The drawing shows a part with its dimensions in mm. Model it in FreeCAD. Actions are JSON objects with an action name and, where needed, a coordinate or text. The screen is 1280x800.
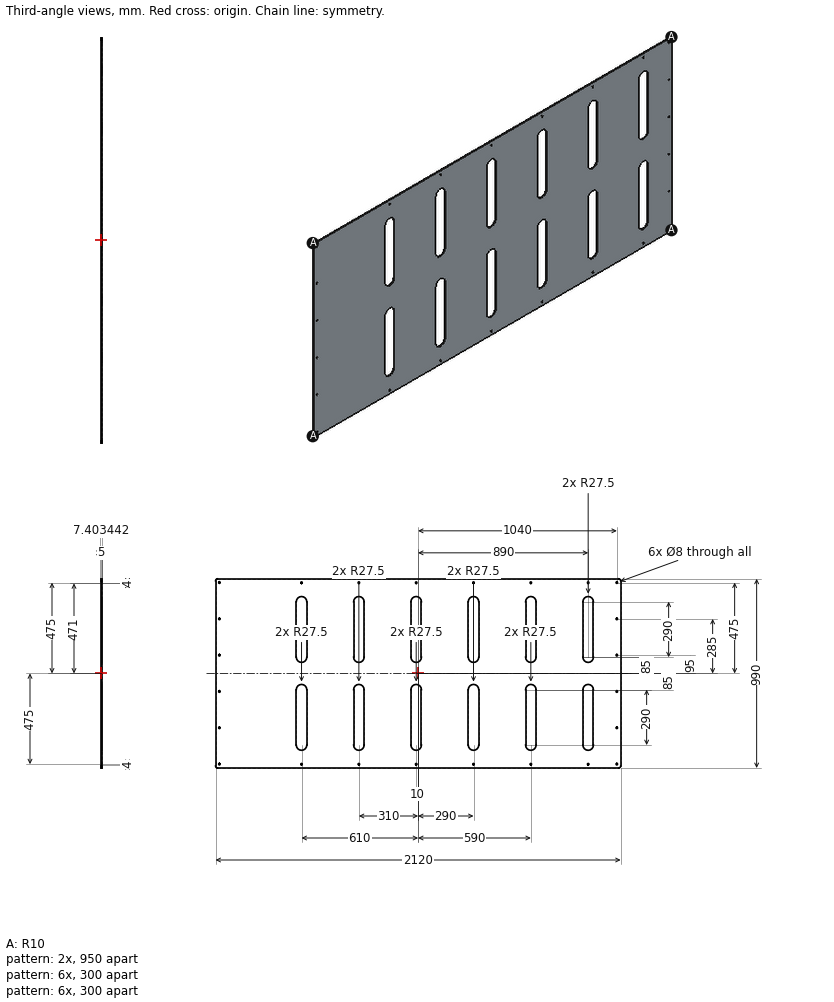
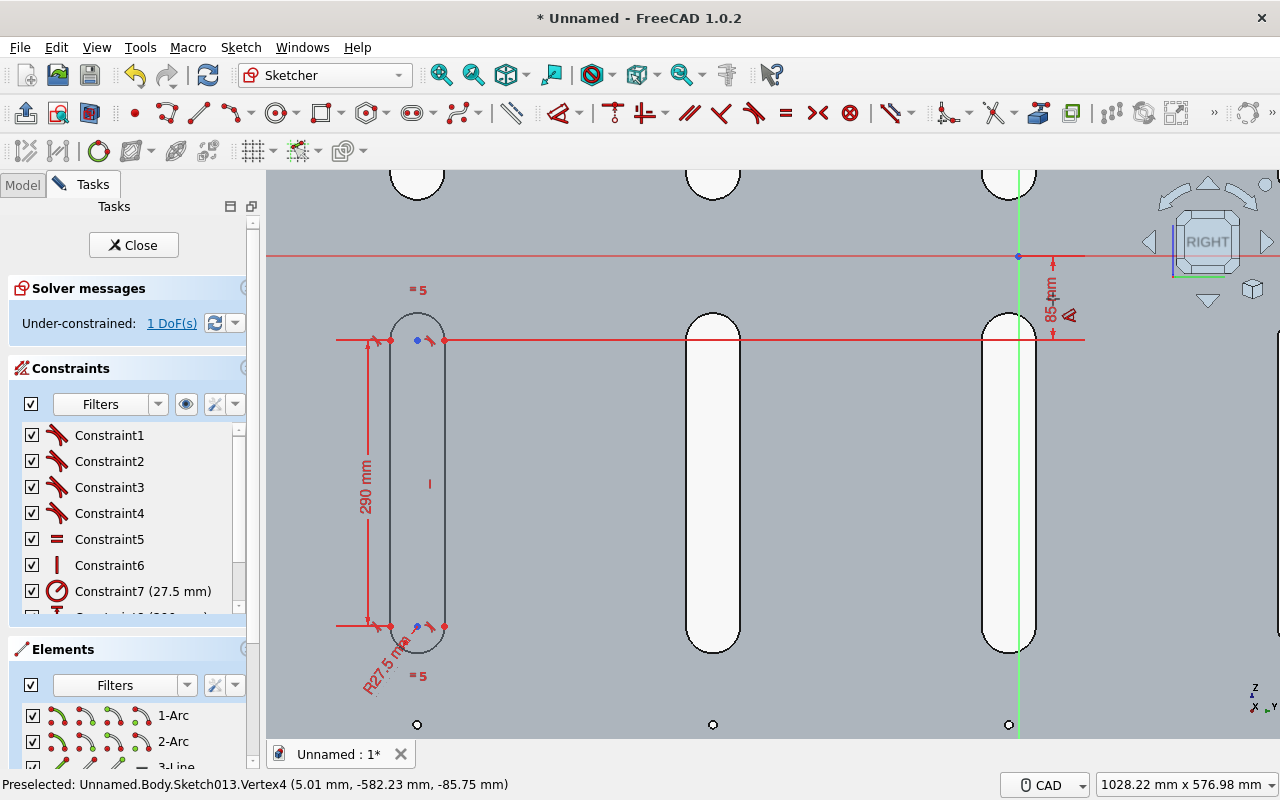
{"action": "left_click", "coordinate": [417, 626]}
{"action": "left_click", "coordinate": [718, 222]}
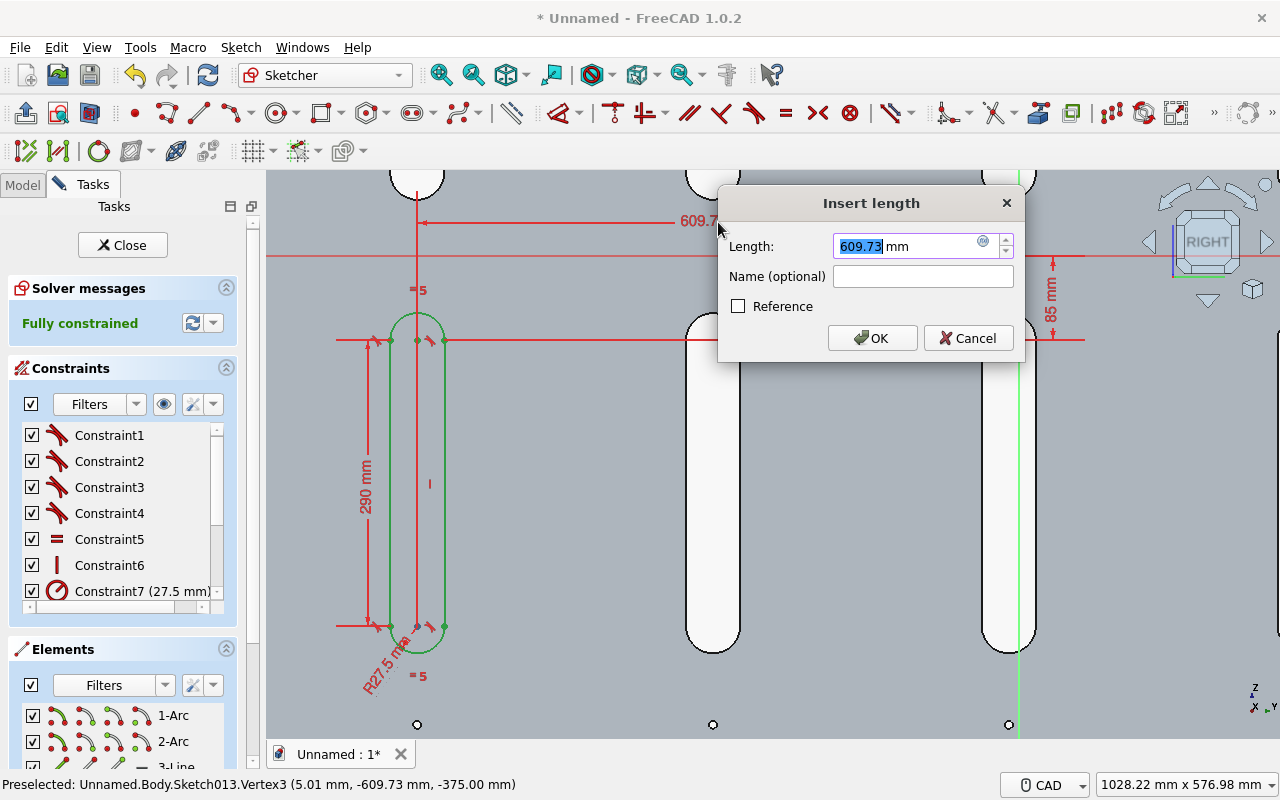
{"action": "type", "text": "610"}
{"action": "key", "text": "Return"}
{"action": "key", "text": "Escape"}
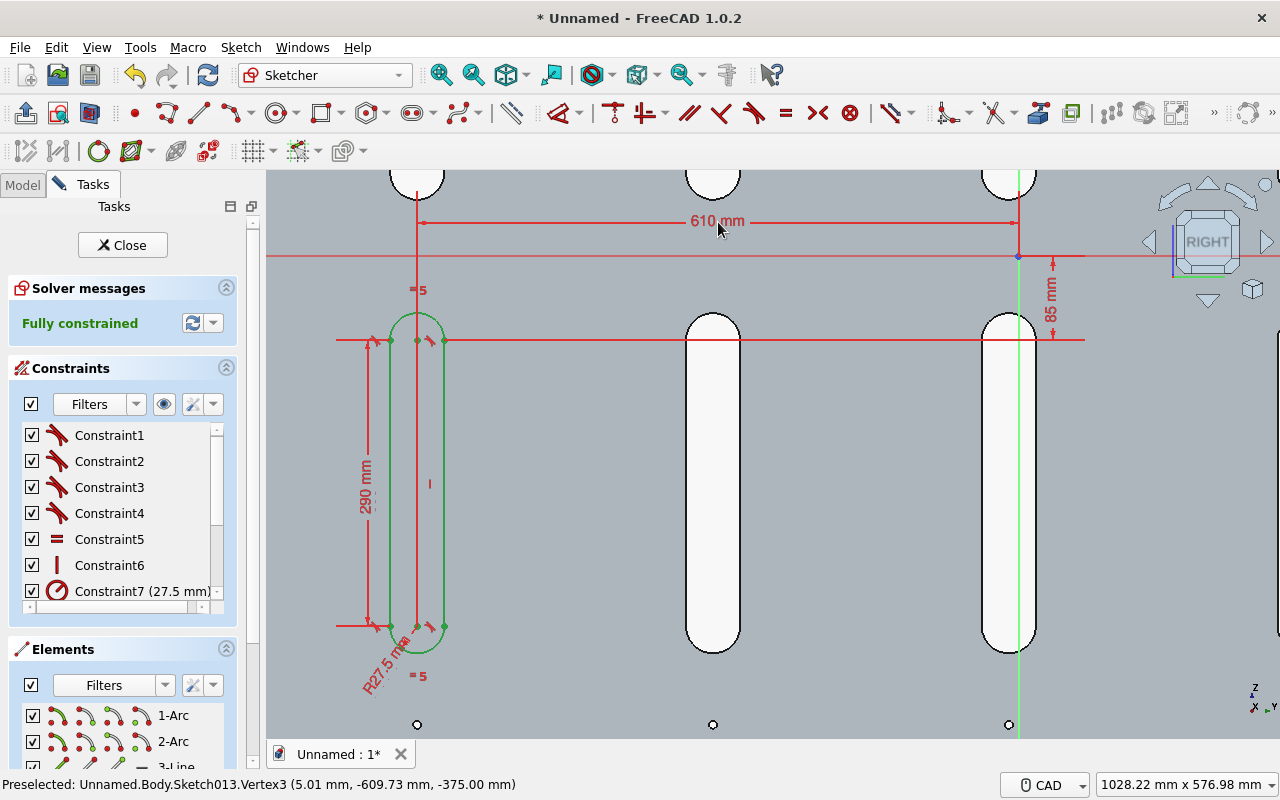
{"action": "left_click", "coordinate": [123, 245]}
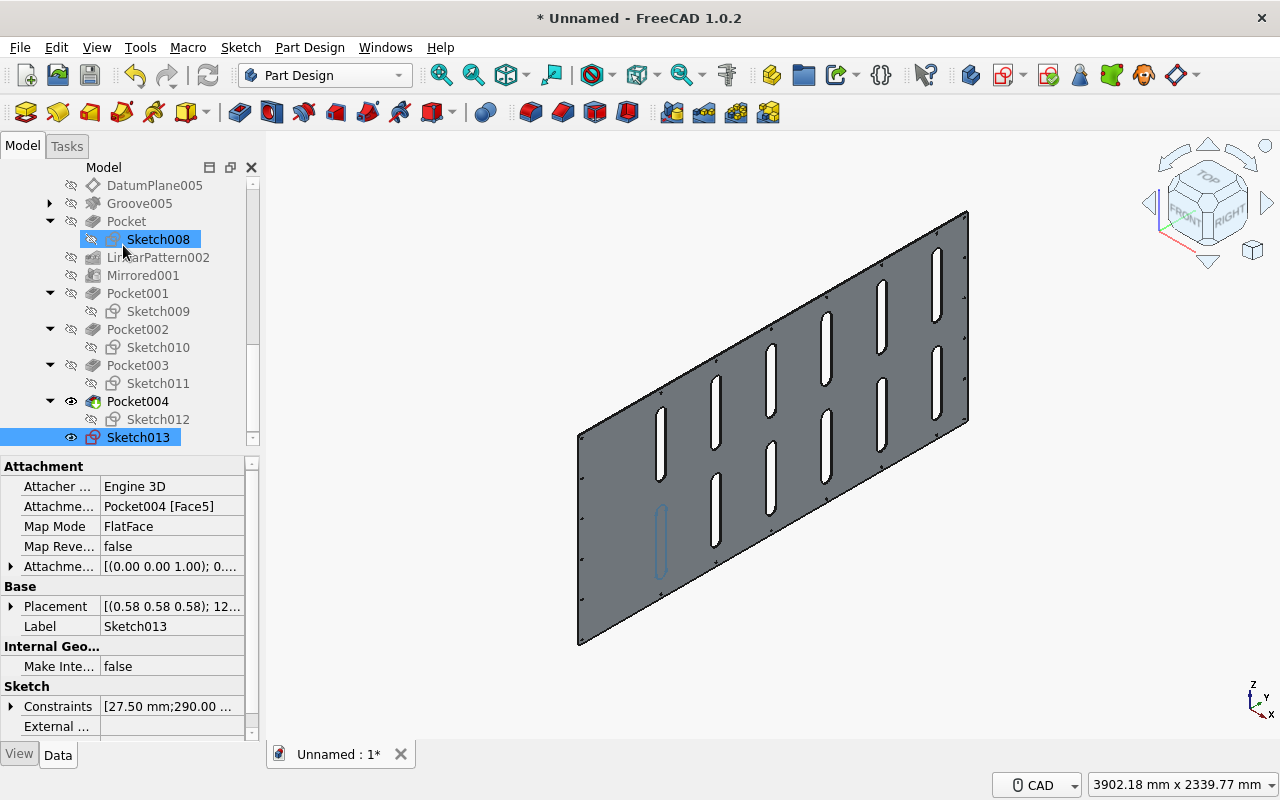
{"action": "left_click", "coordinate": [240, 112]}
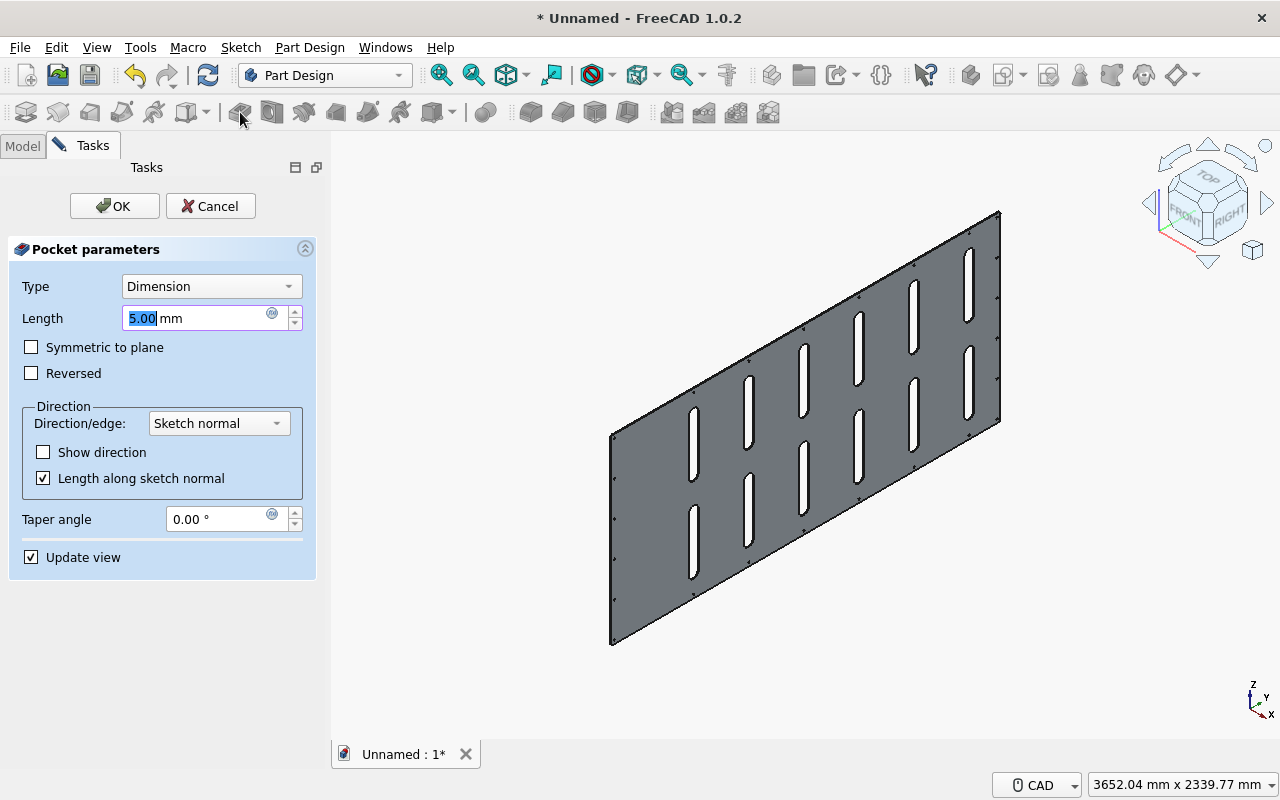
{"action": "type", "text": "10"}
{"action": "key", "text": "Tab"}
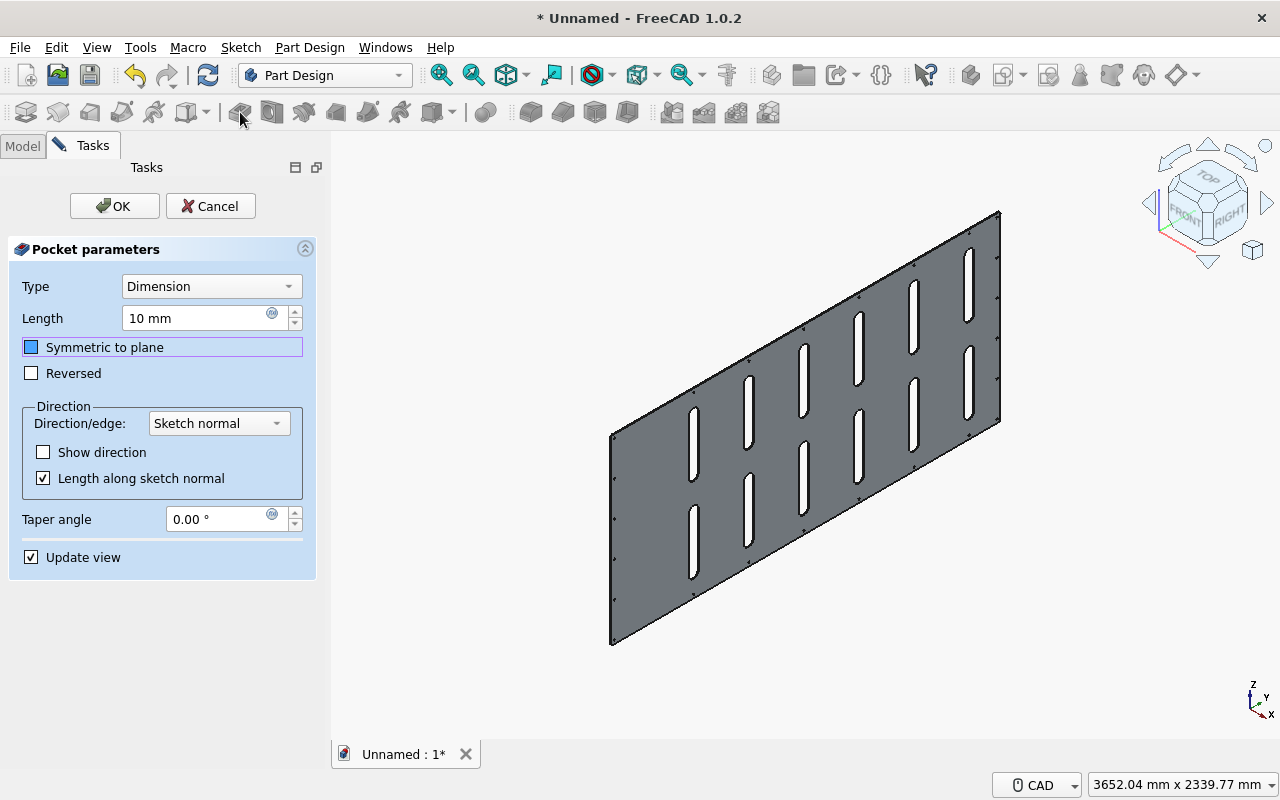
{"action": "left_click", "coordinate": [115, 206]}